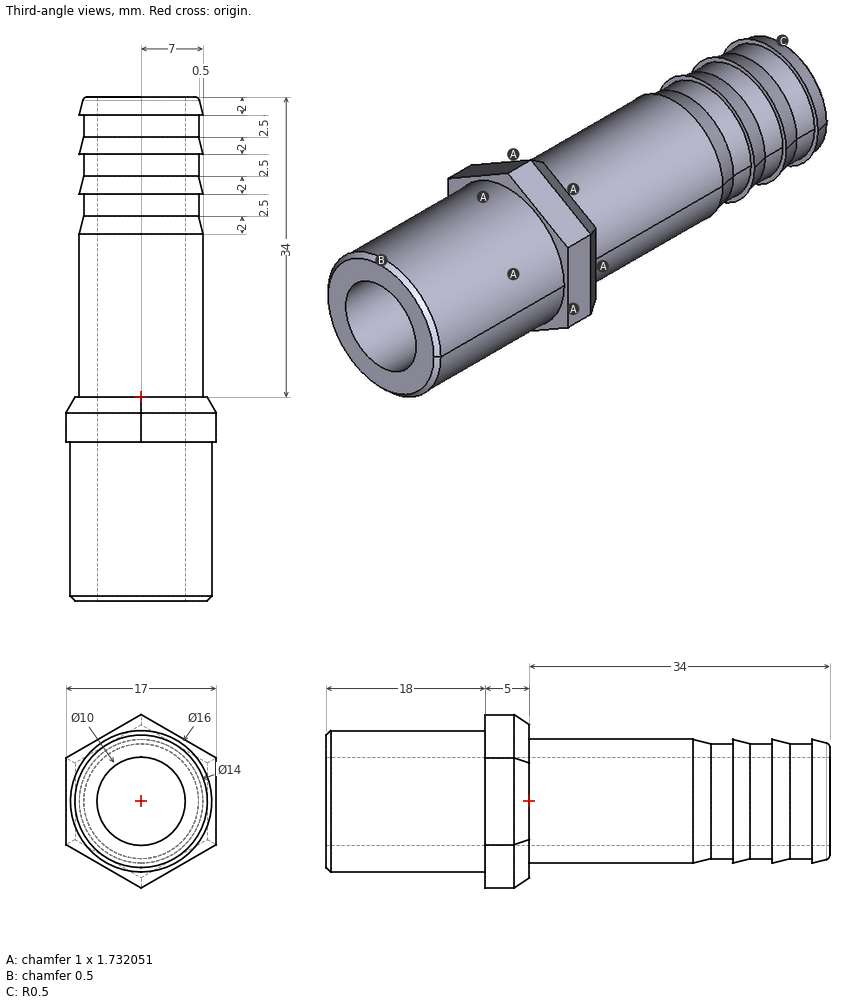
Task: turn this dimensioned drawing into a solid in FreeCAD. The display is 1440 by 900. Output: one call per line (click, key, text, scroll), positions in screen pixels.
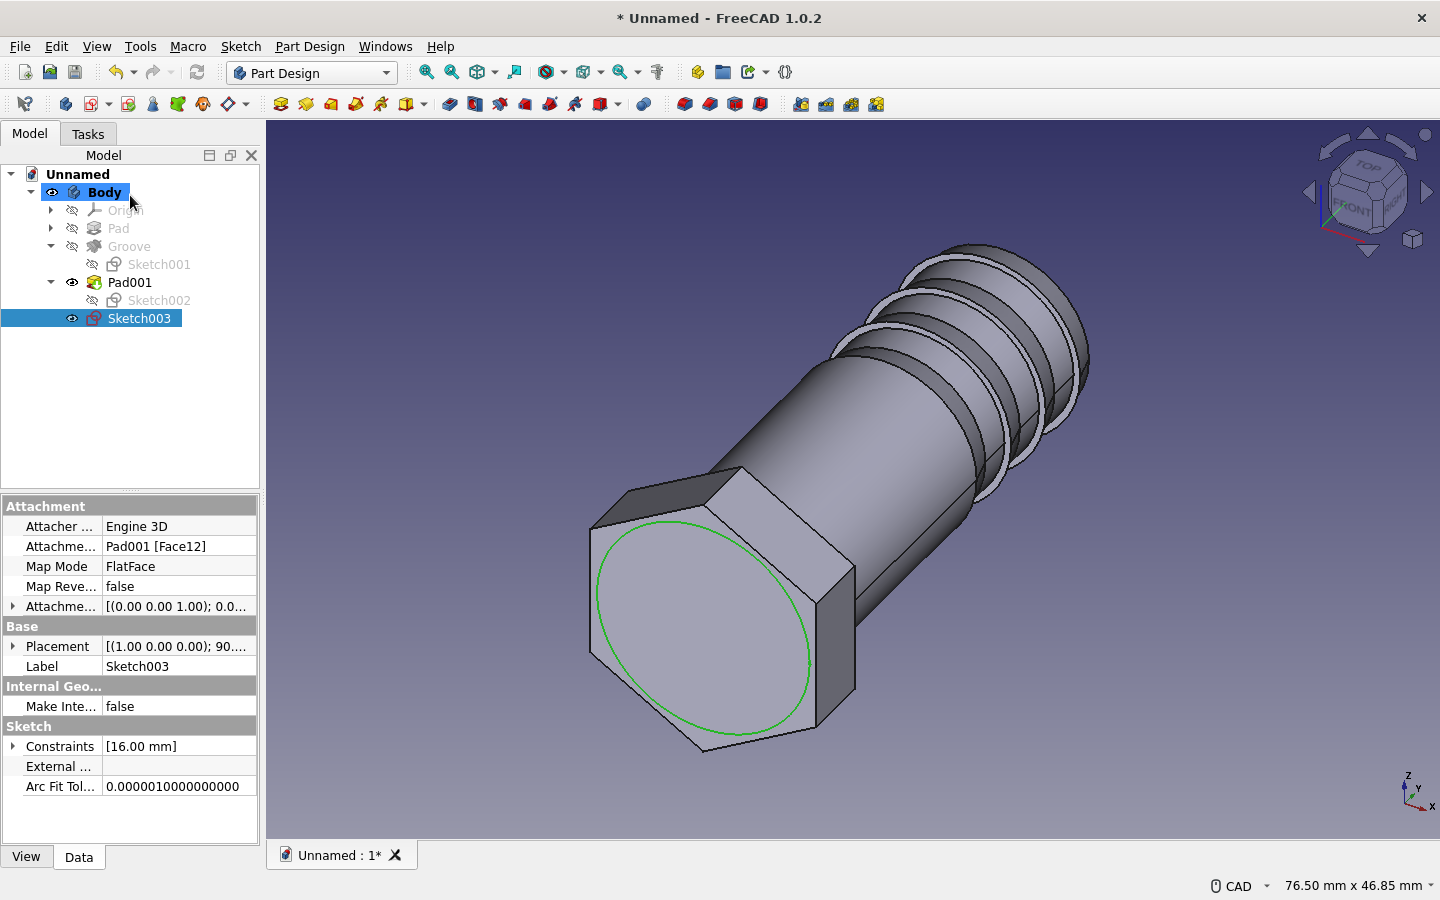
click(281, 104)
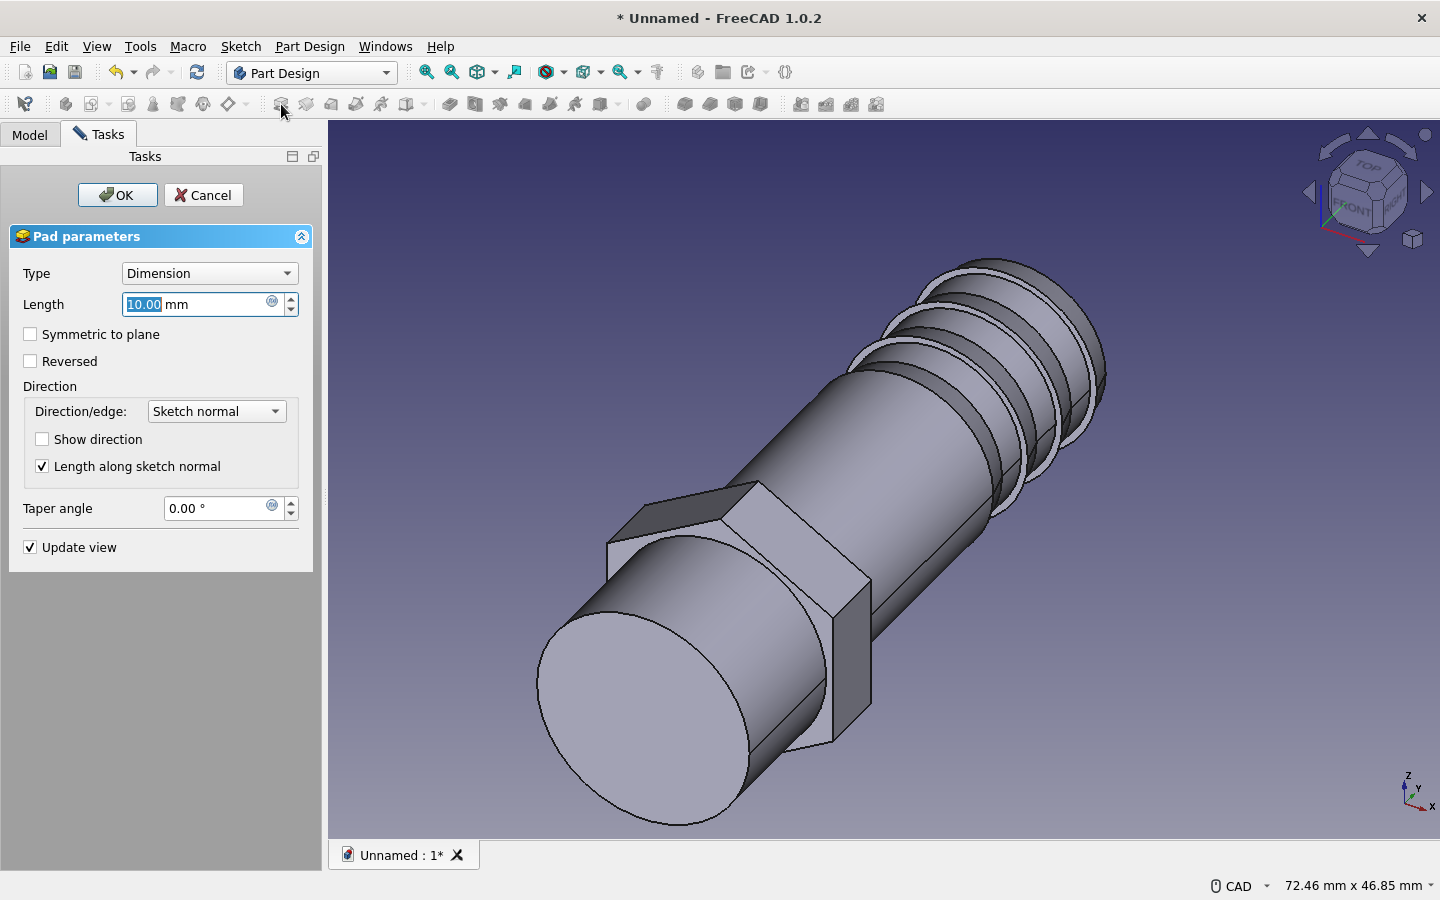
text(18)
key(Tab)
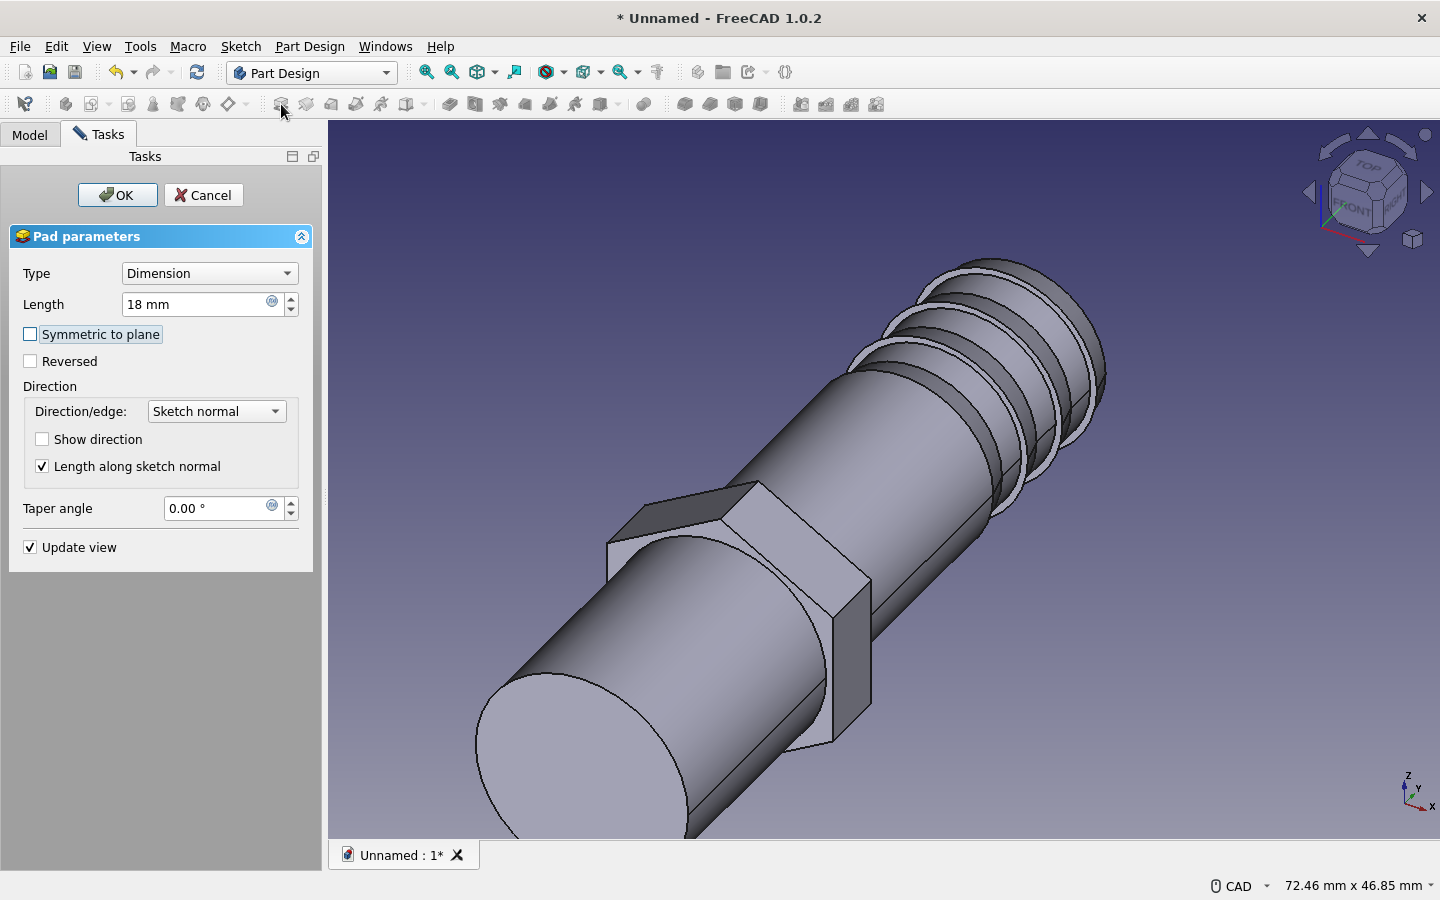
click(118, 195)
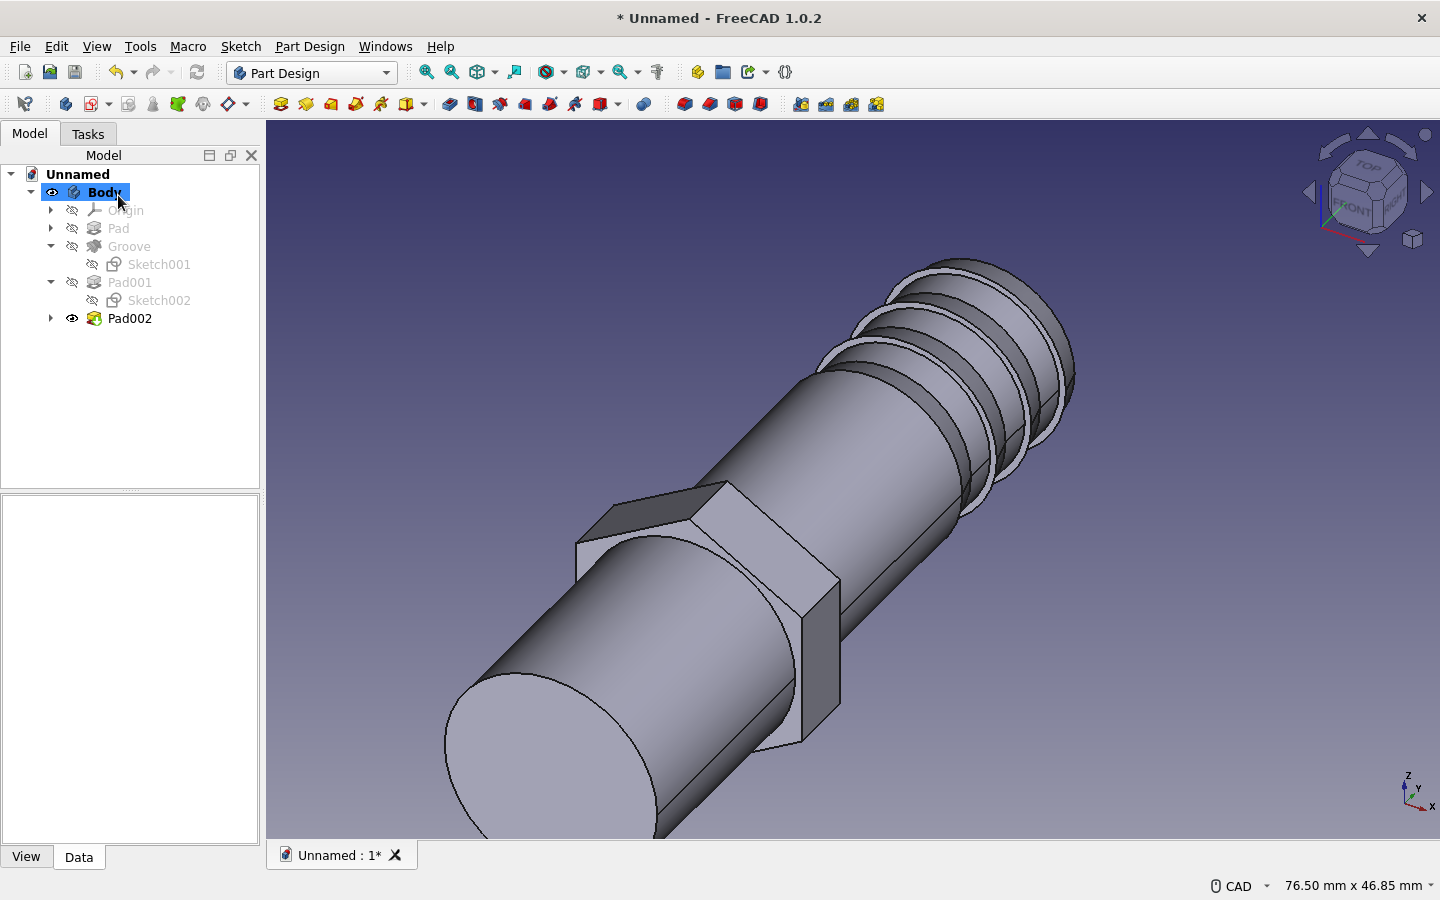
click(427, 72)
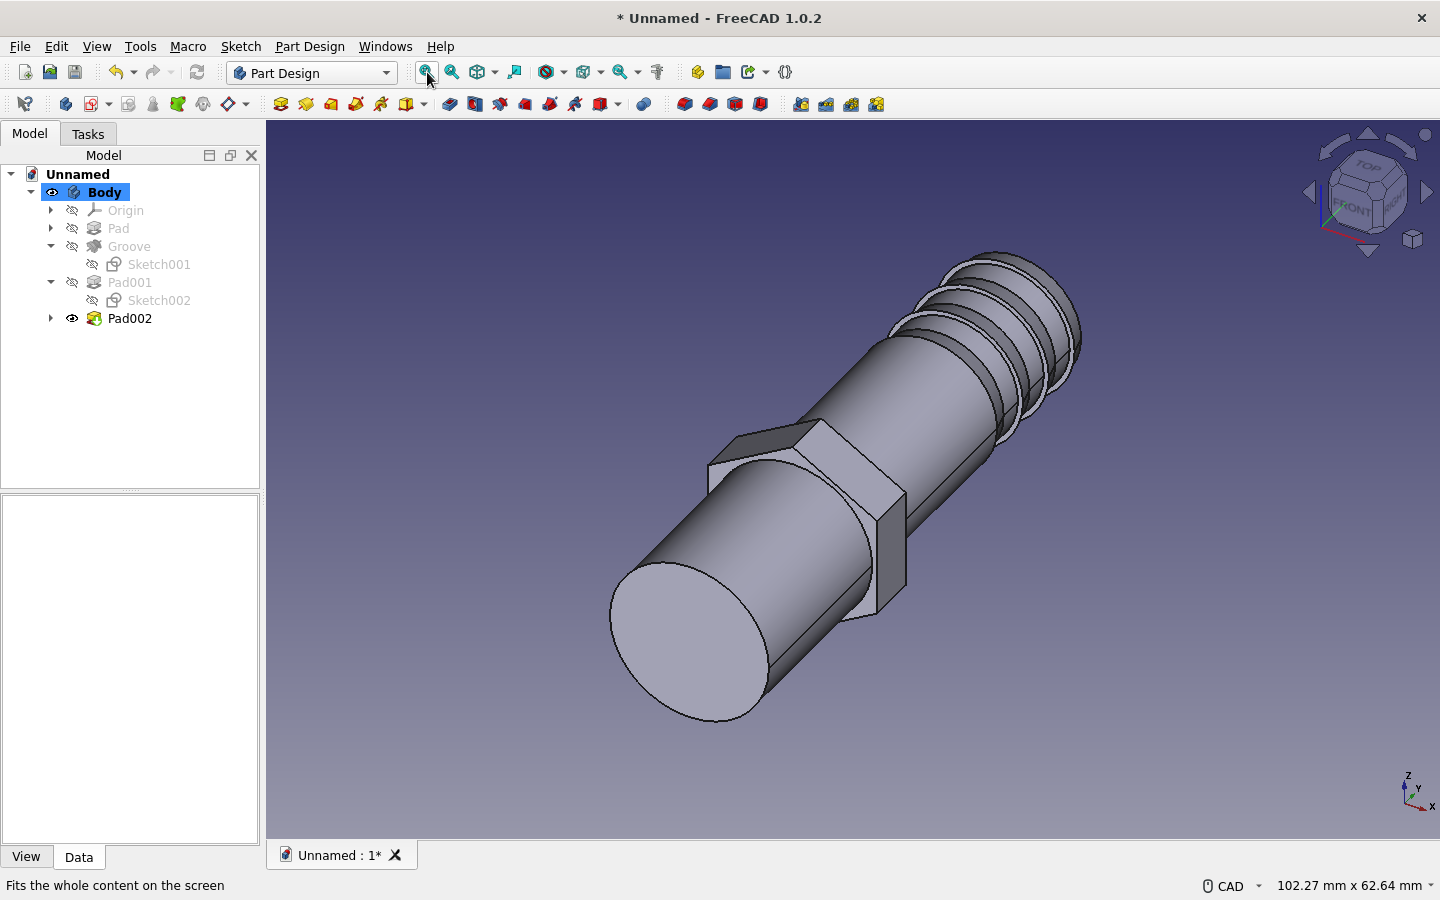
key(4)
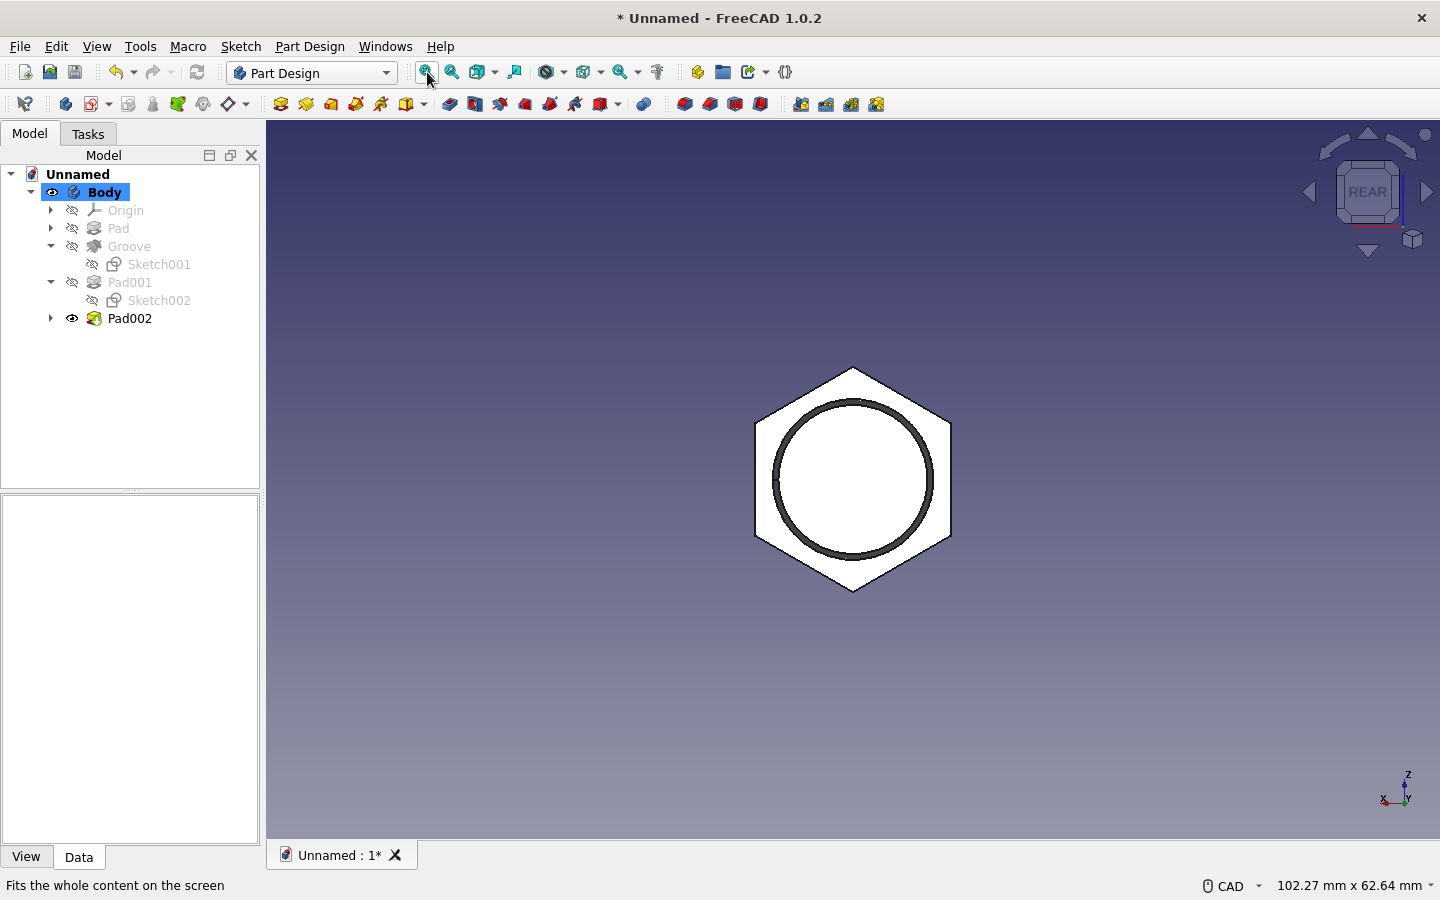
click(427, 72)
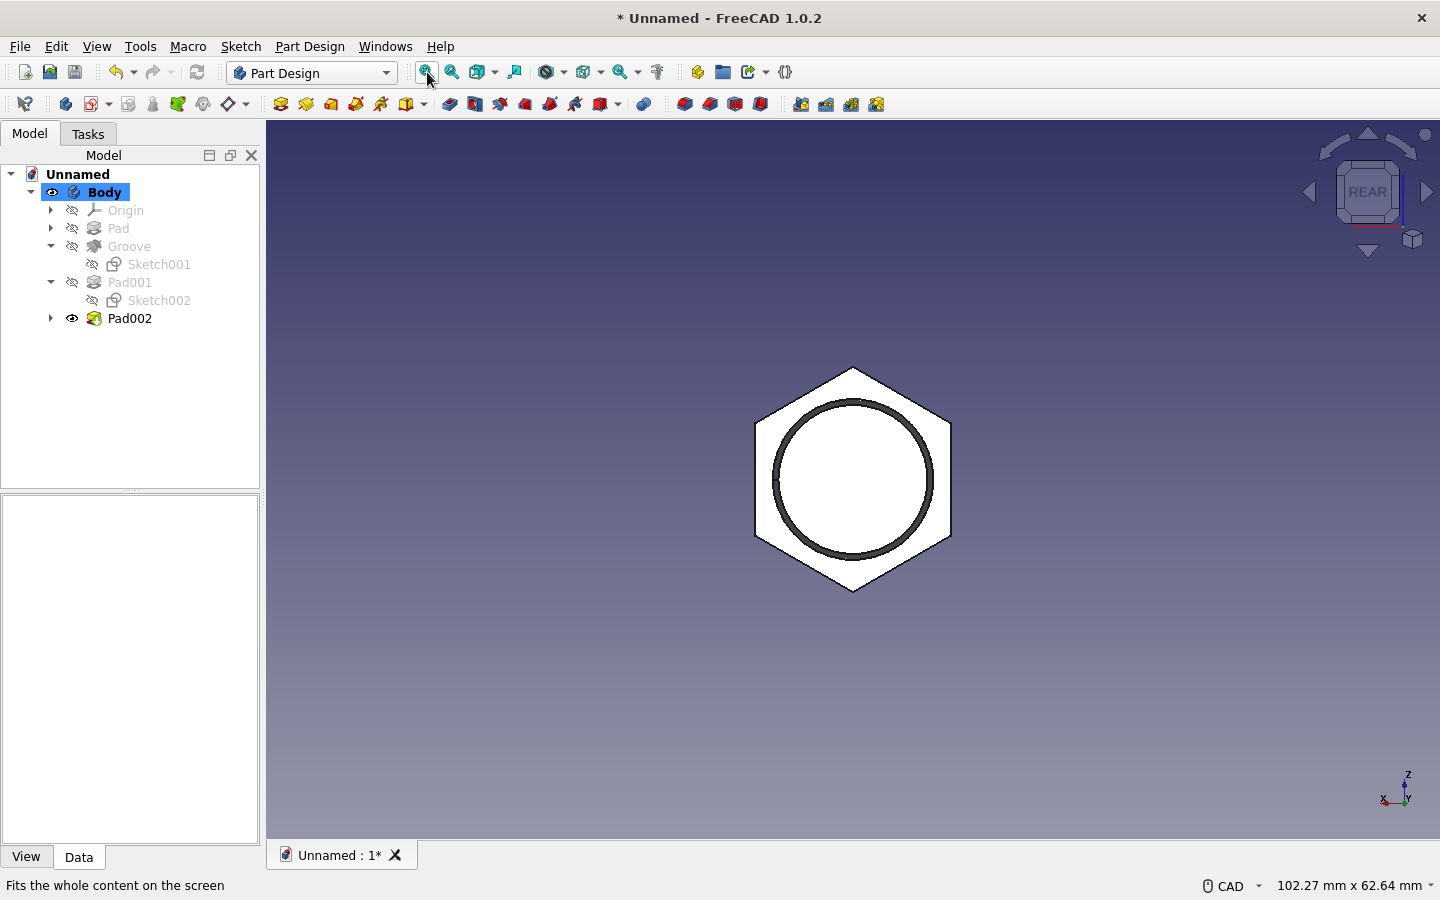
click(853, 479)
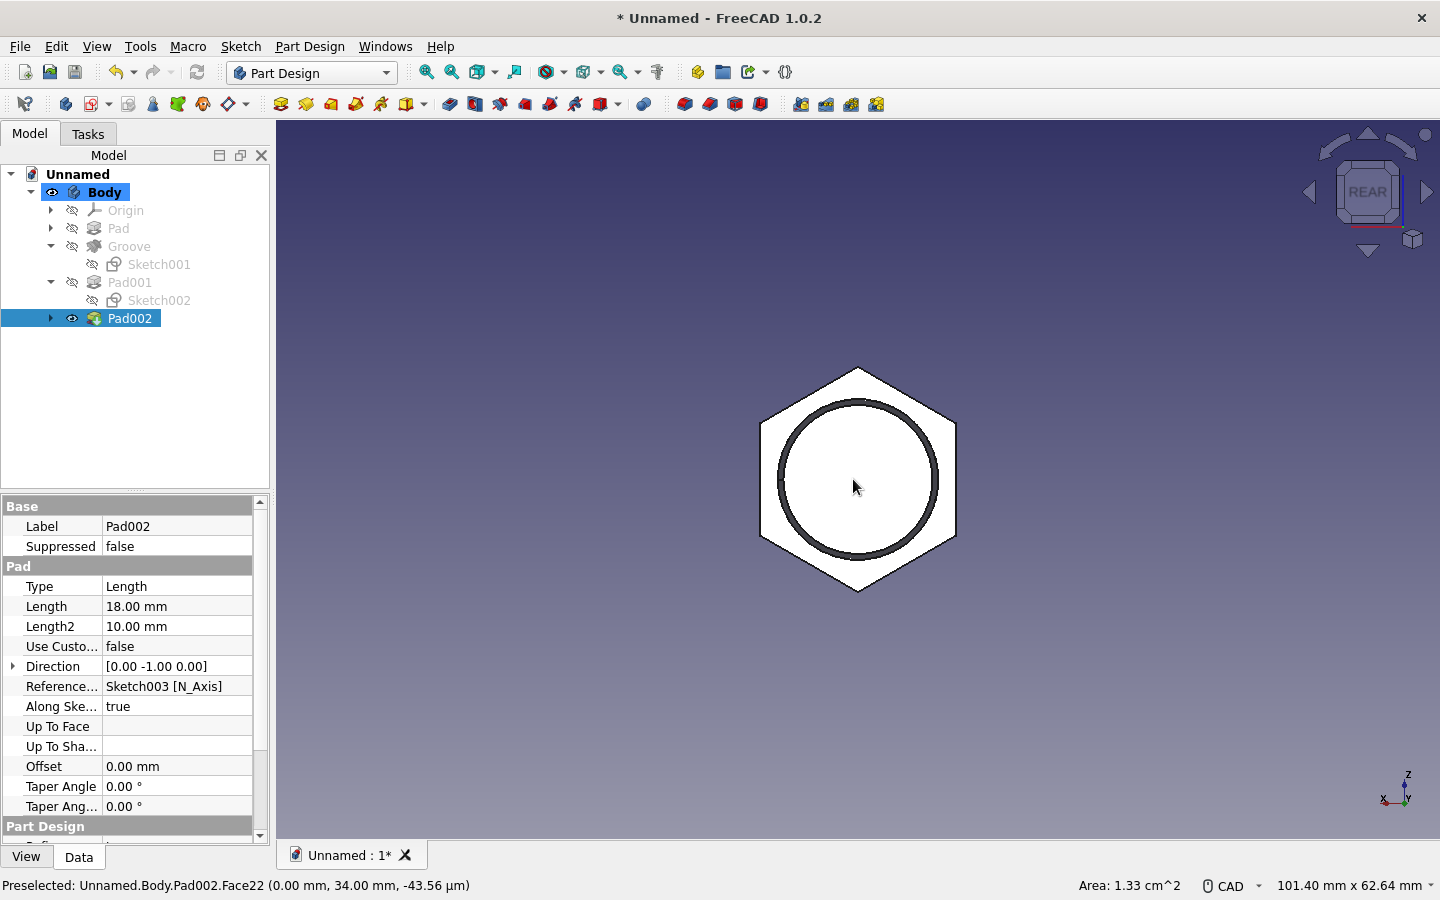
click(90, 104)